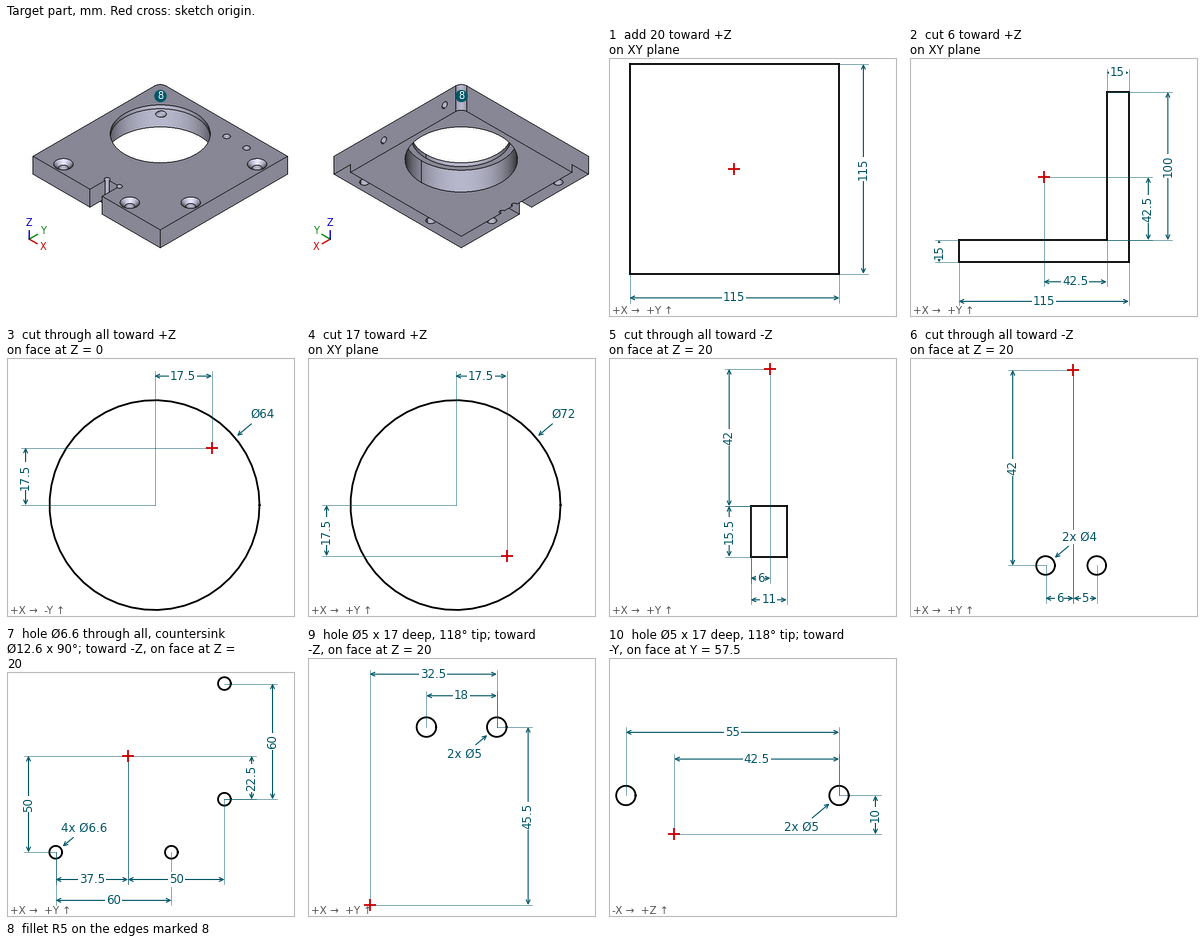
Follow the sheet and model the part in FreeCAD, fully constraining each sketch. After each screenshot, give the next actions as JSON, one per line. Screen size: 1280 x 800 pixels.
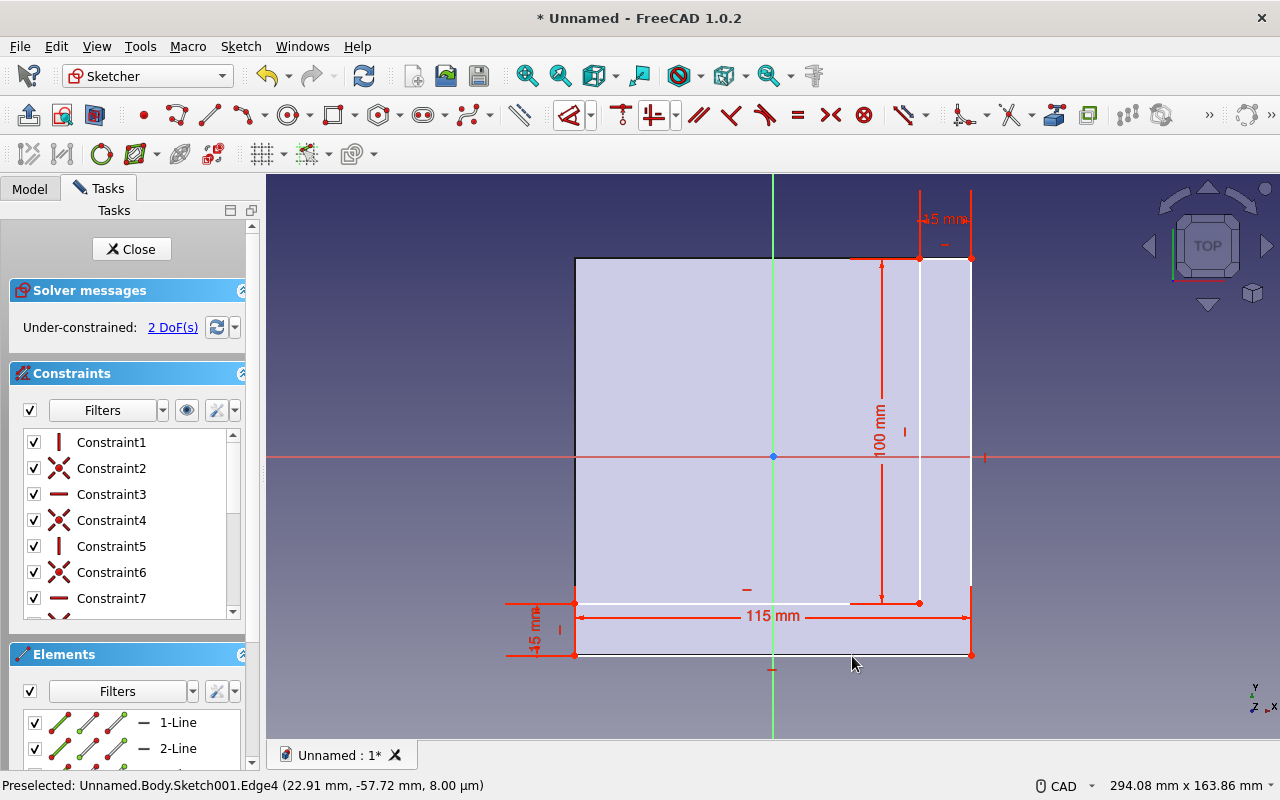
{"action": "left_click", "coordinate": [920, 604]}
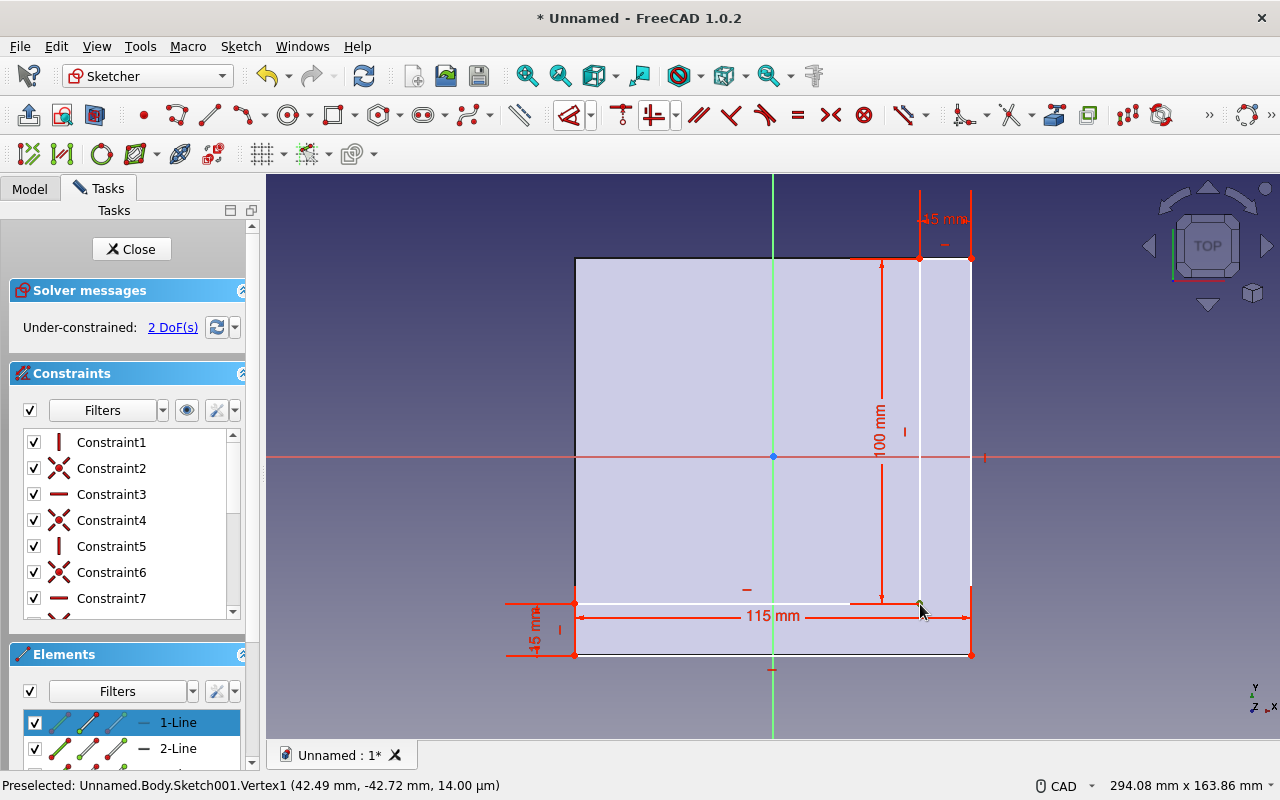
{"action": "key", "text": "l"}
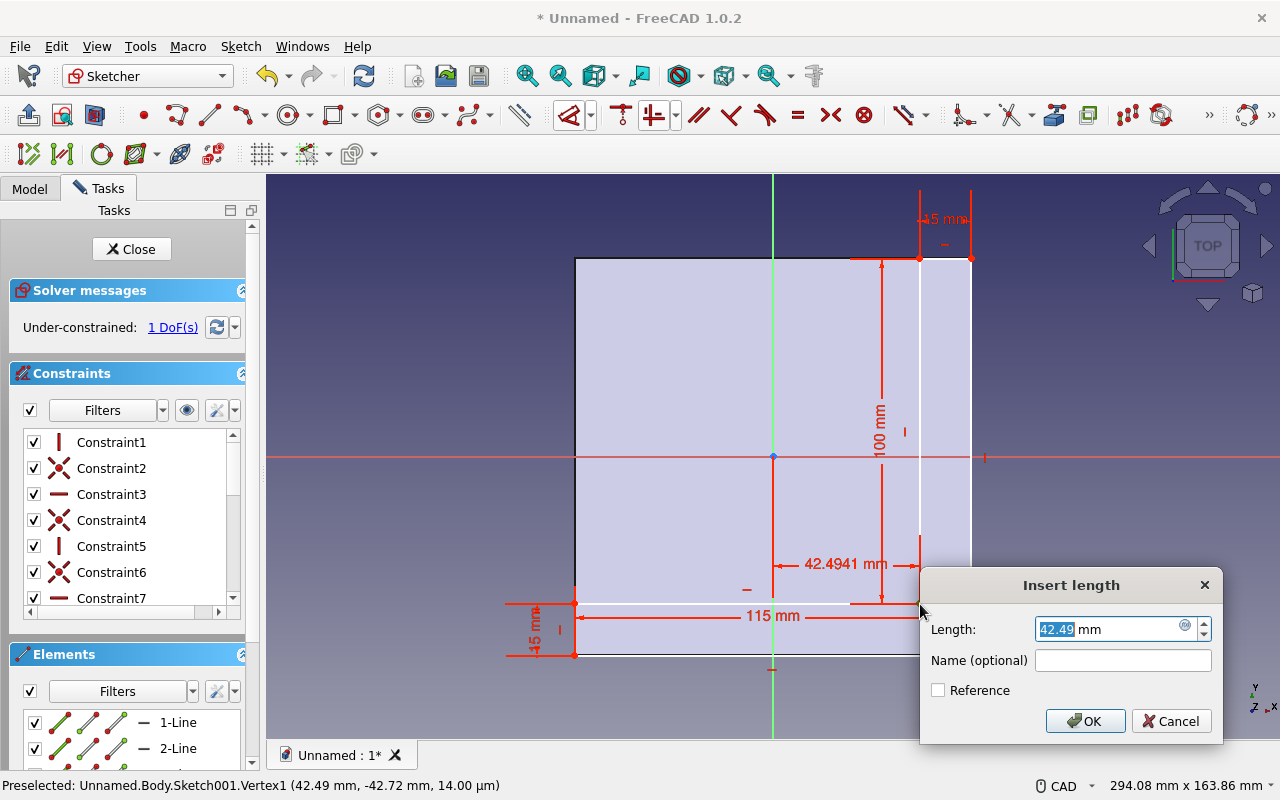
{"action": "type", "text": "42.5"}
{"action": "key", "text": "Return"}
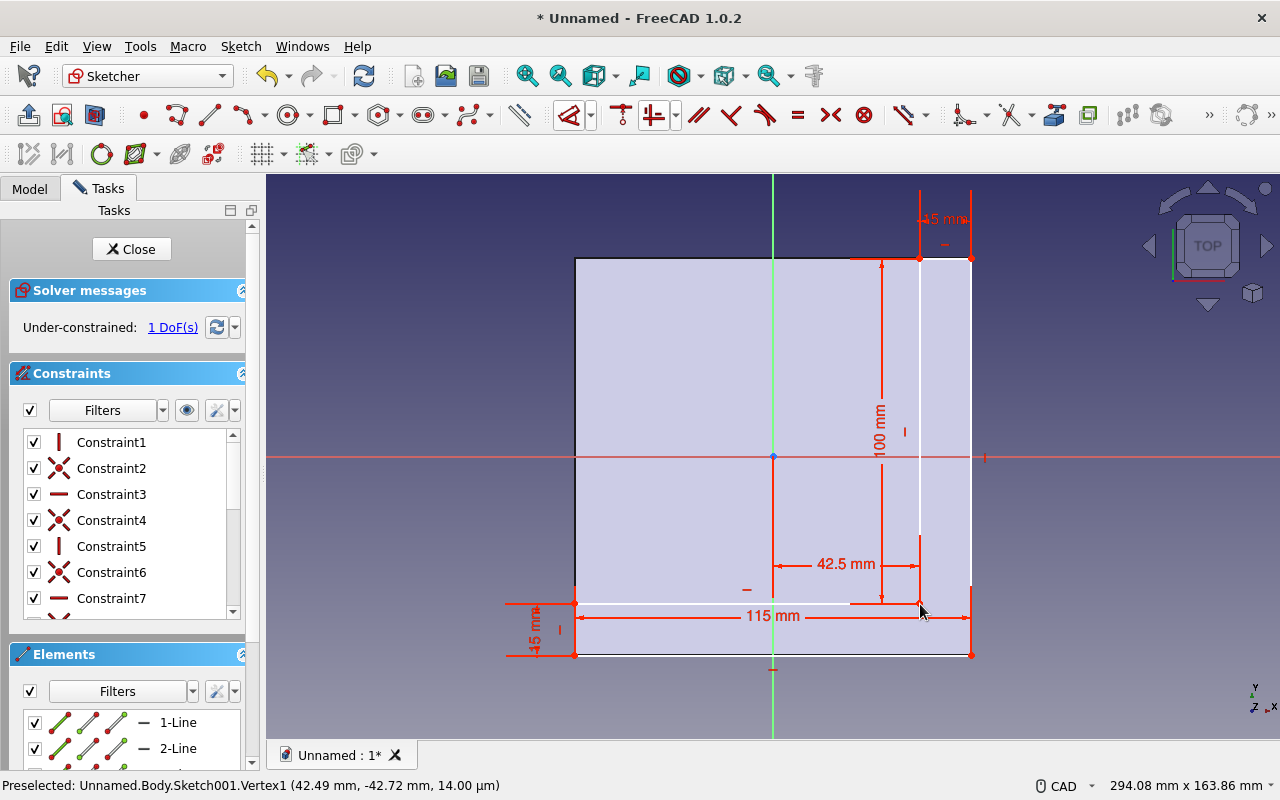
{"action": "left_click", "coordinate": [920, 604]}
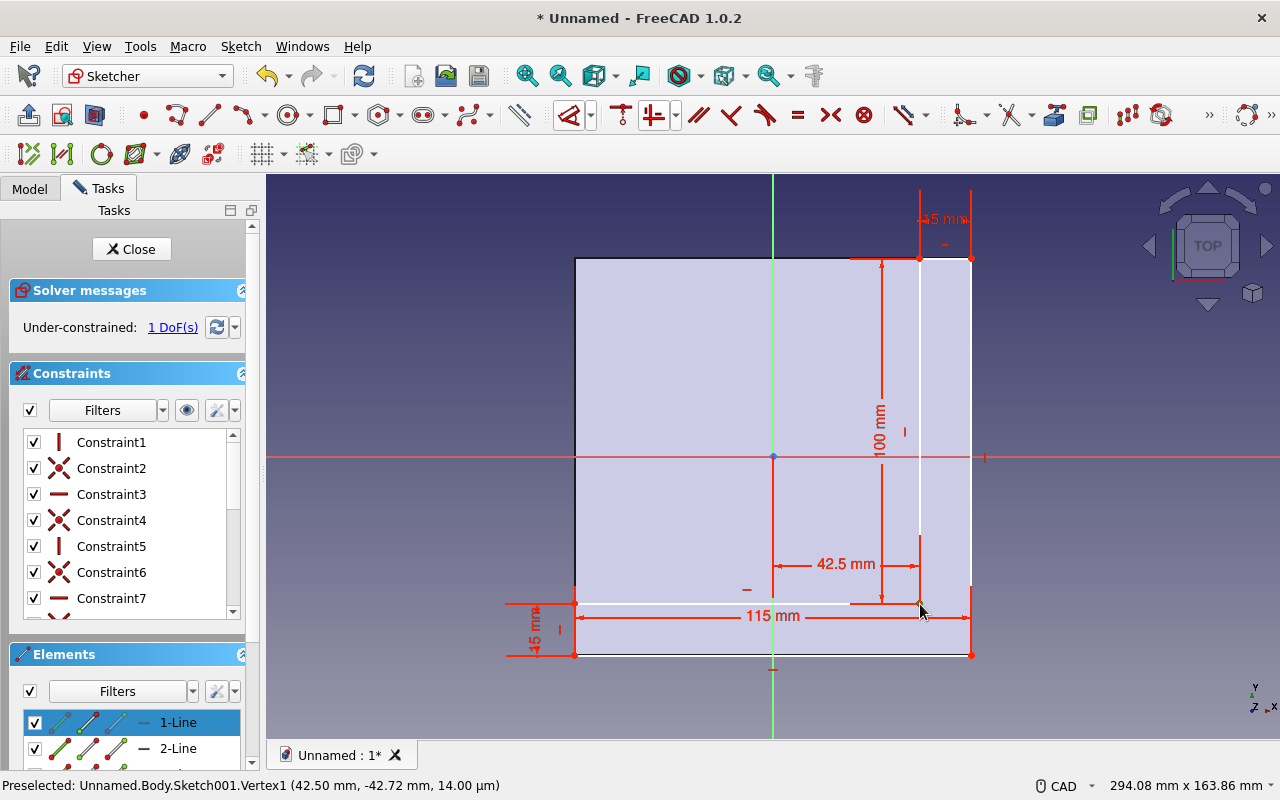
{"action": "key", "text": "i"}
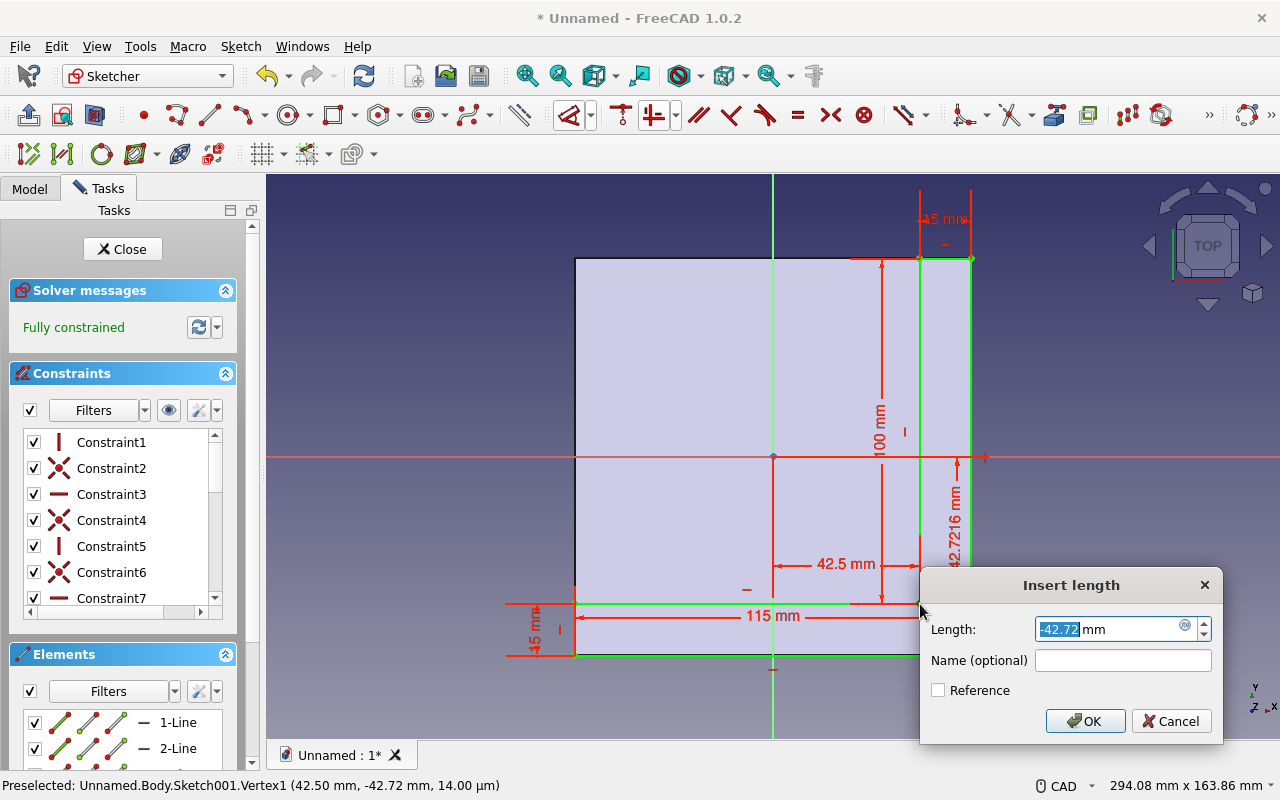
{"action": "type", "text": "-42.5"}
{"action": "key", "text": "Return"}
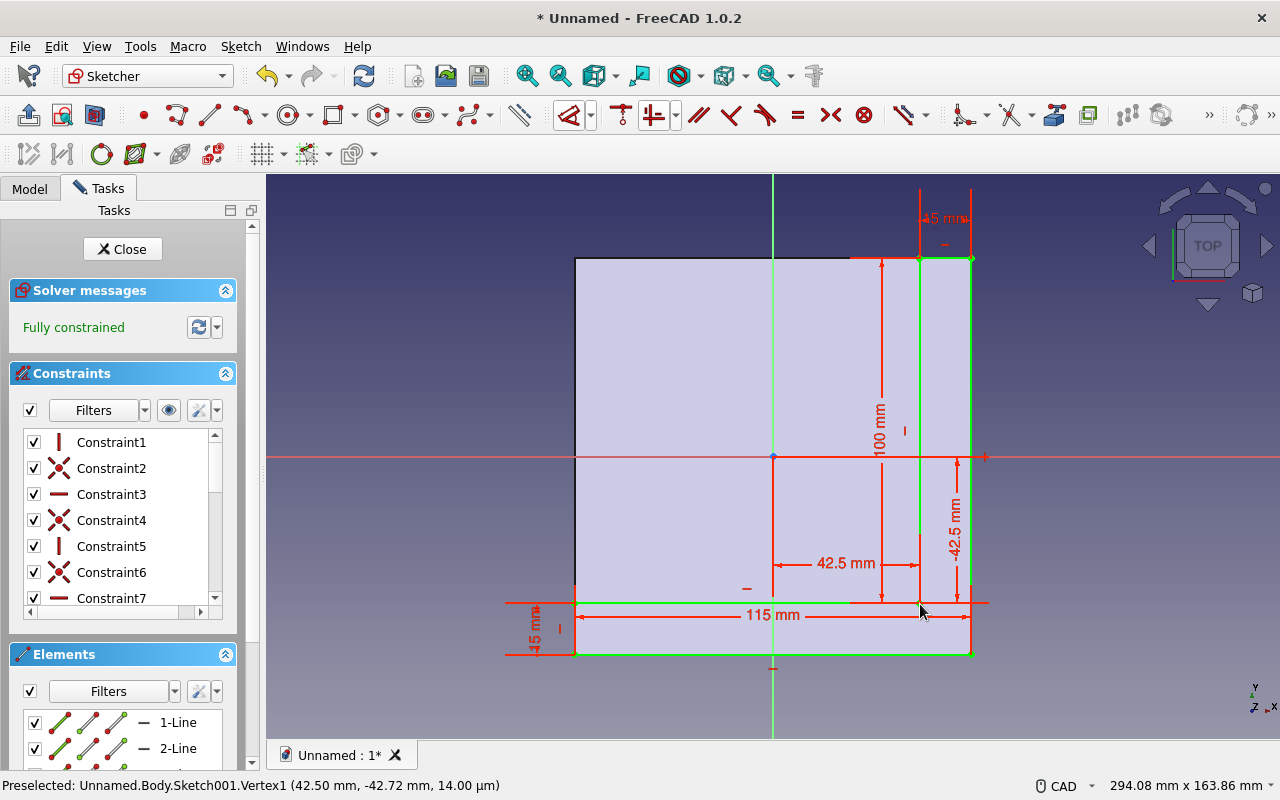
{"action": "left_click", "coordinate": [123, 249]}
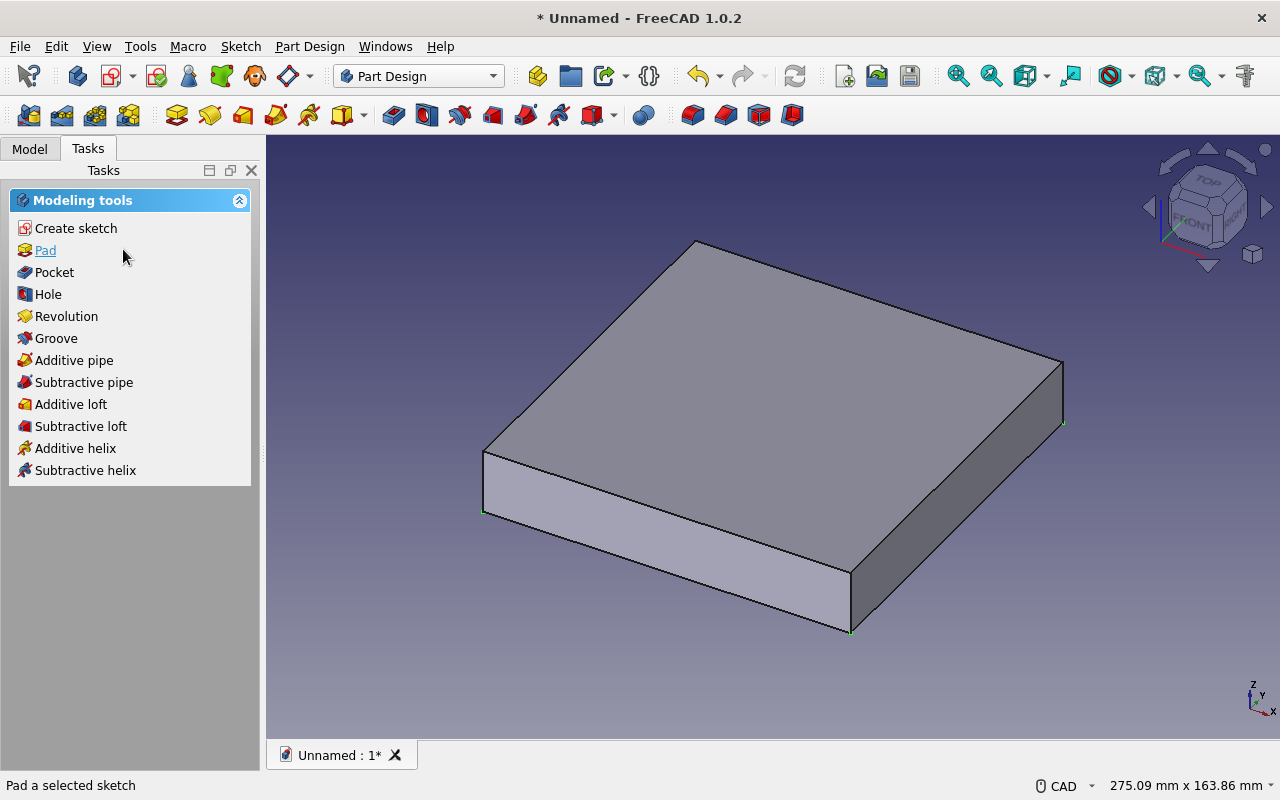
{"action": "left_click", "coordinate": [394, 116]}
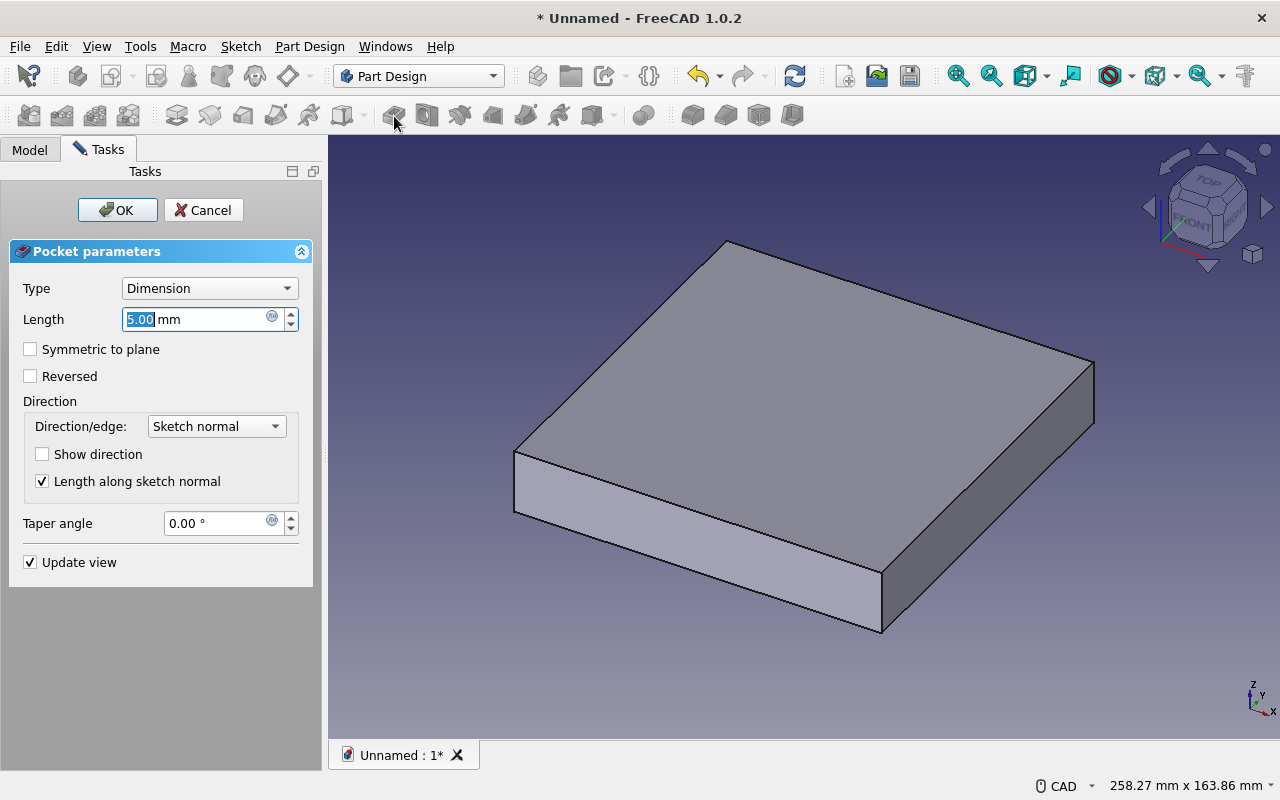
{"action": "type", "text": "6"}
{"action": "key", "text": "Tab"}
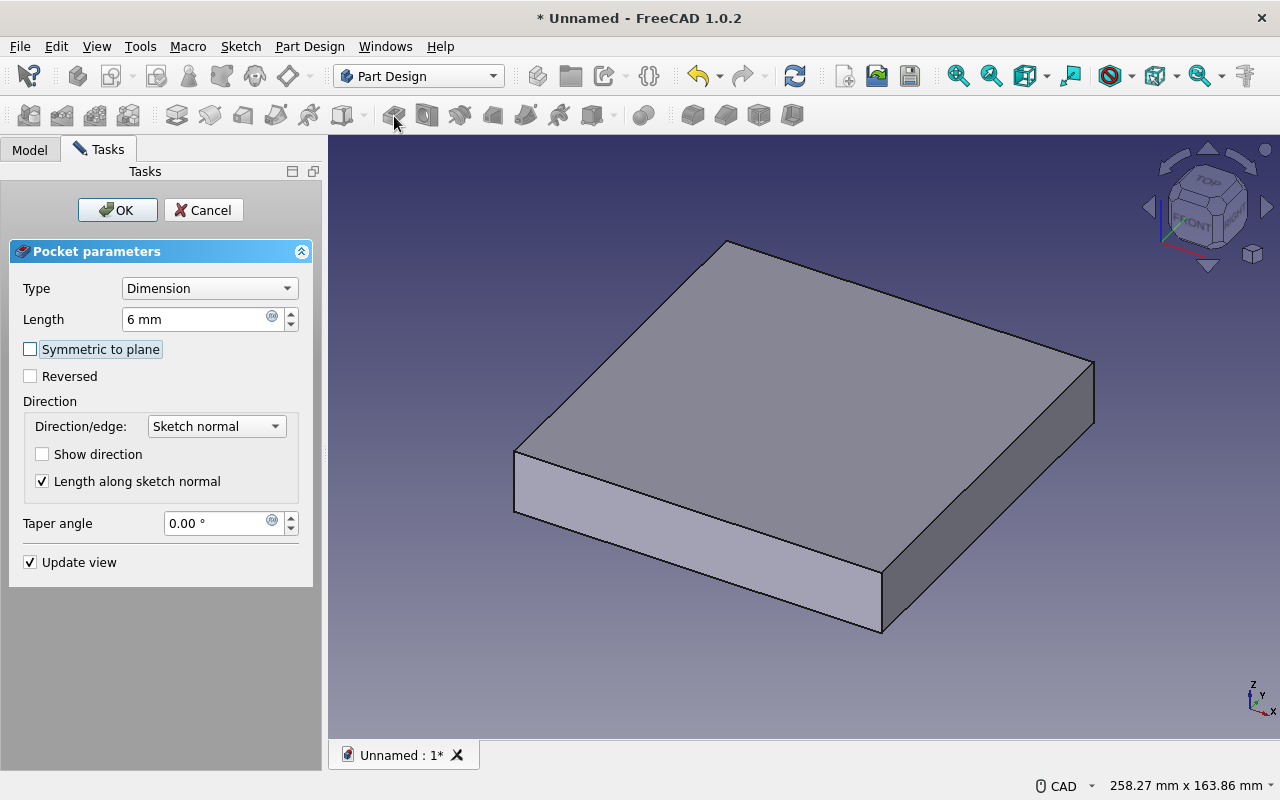
{"action": "left_click", "coordinate": [31, 376]}